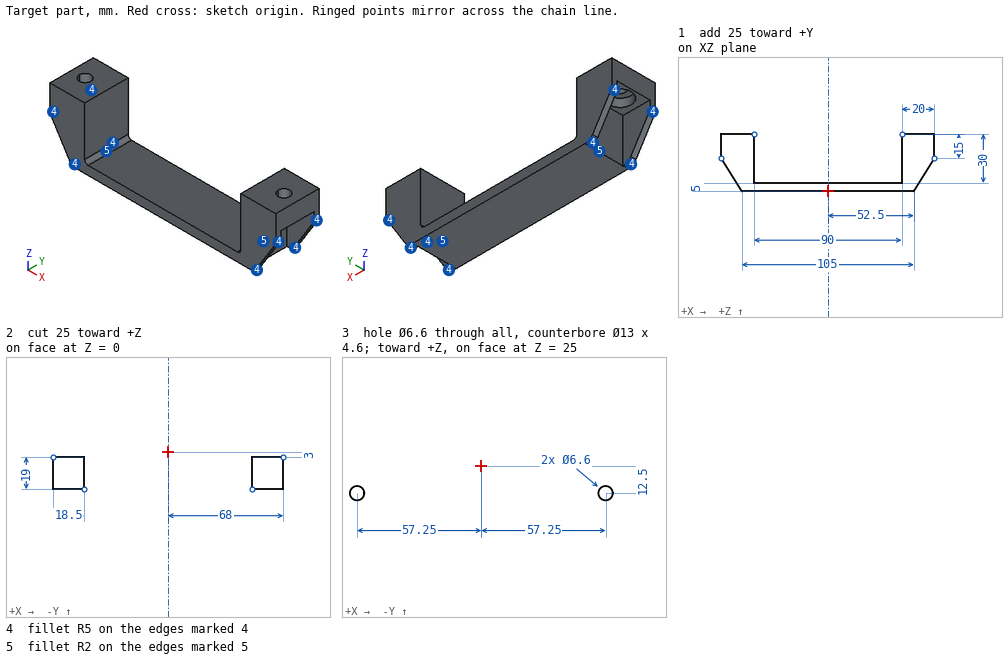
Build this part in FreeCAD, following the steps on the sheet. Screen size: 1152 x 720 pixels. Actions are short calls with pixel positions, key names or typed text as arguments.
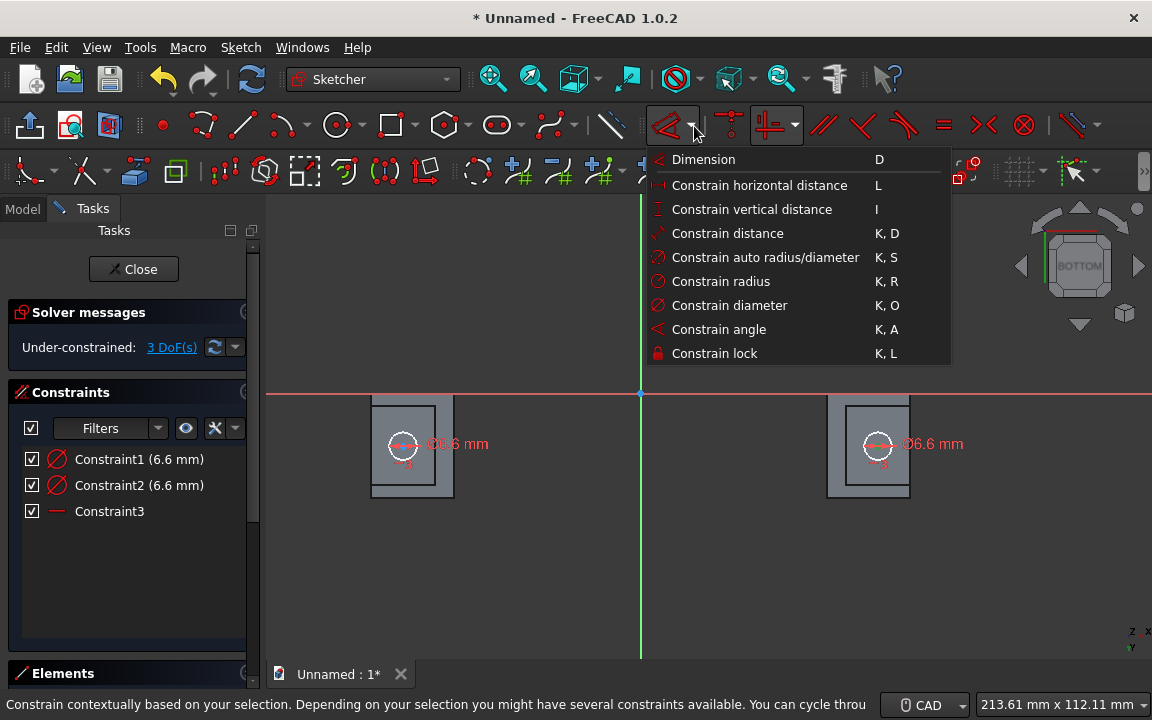
click(799, 209)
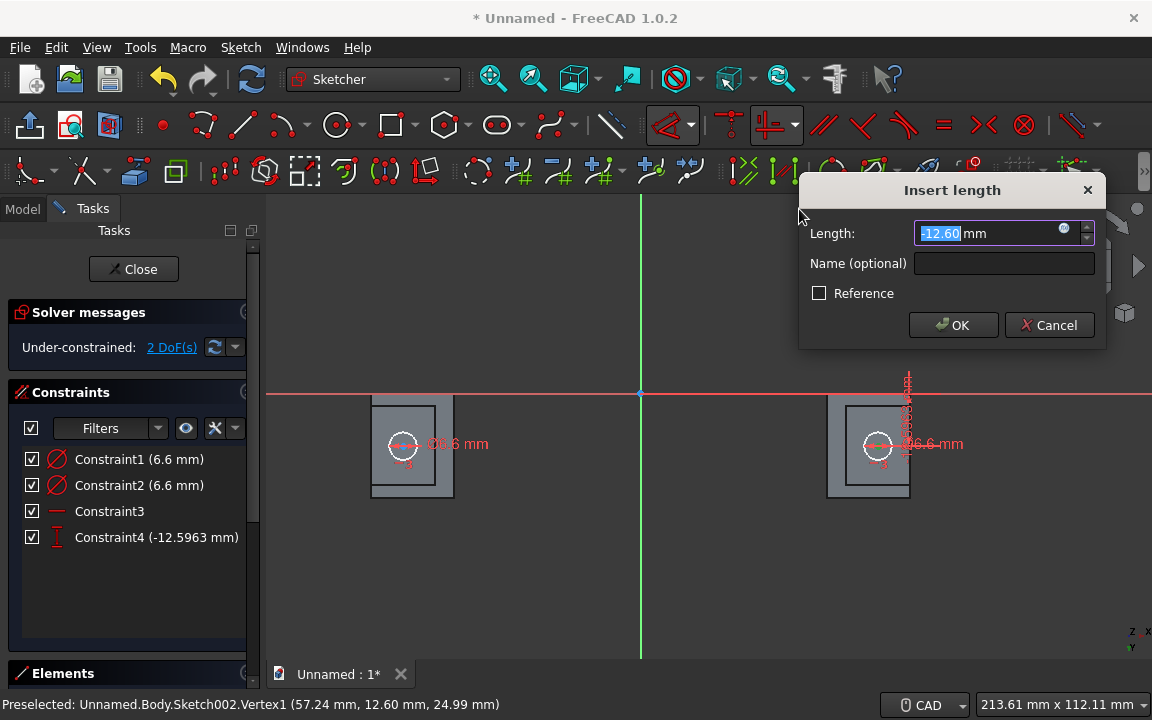
text(-12.5)
key(Return)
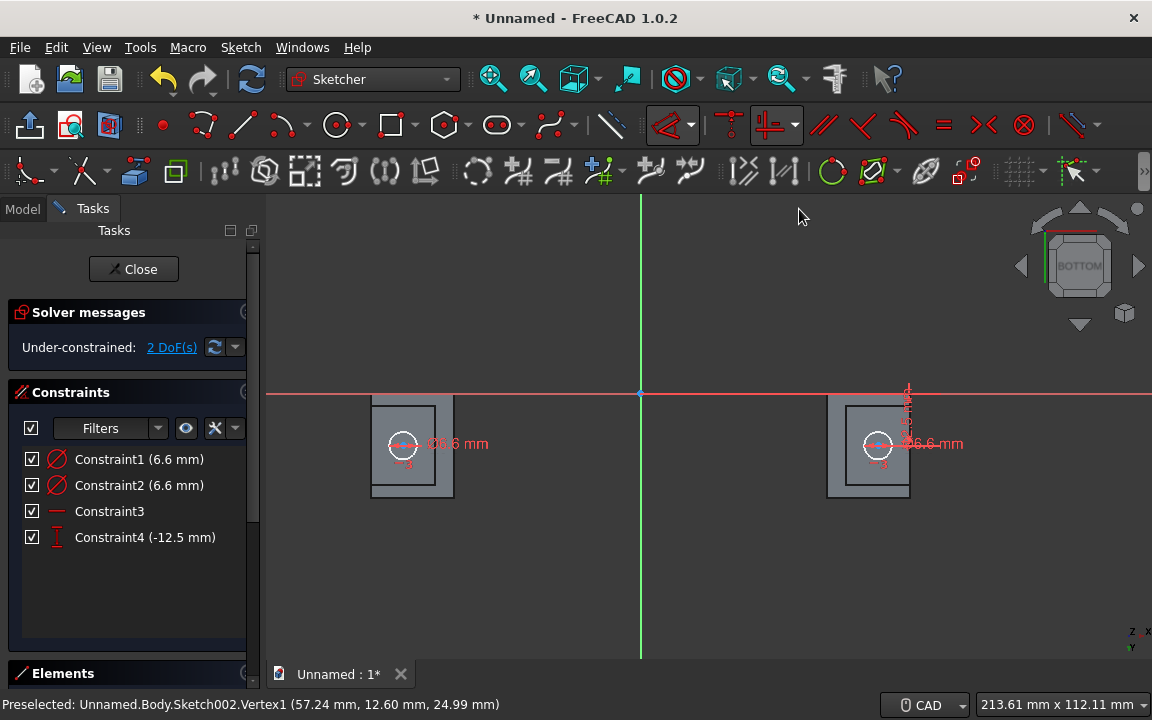
click(878, 446)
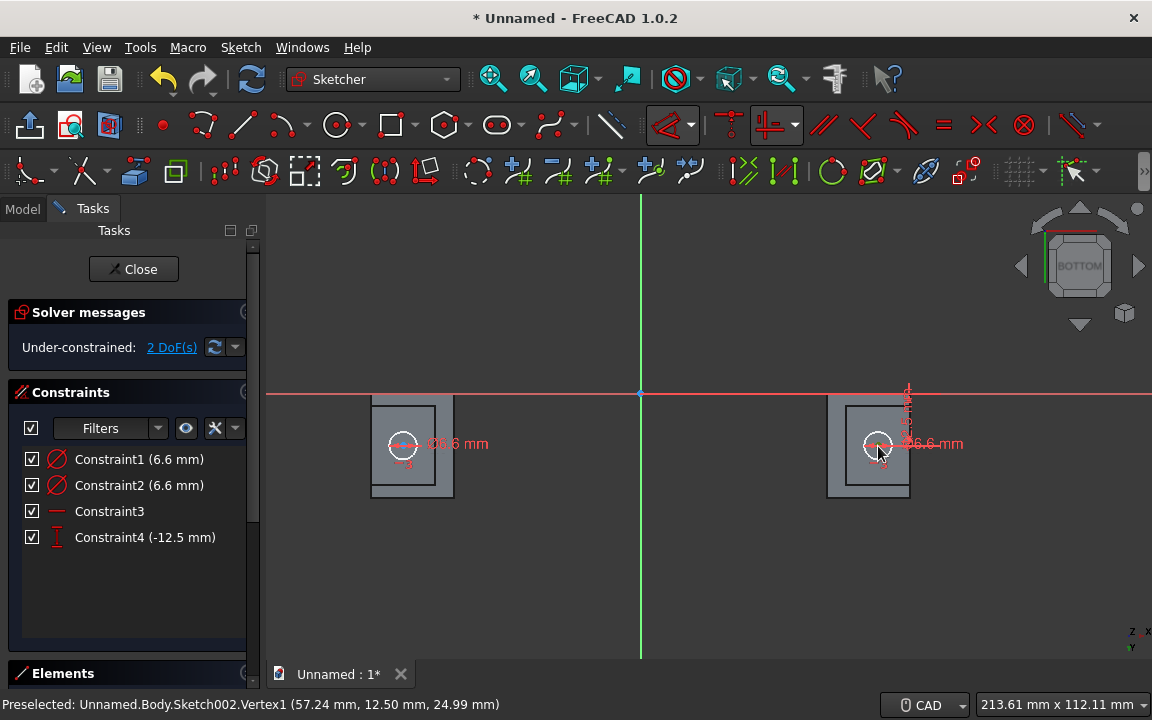
key(l)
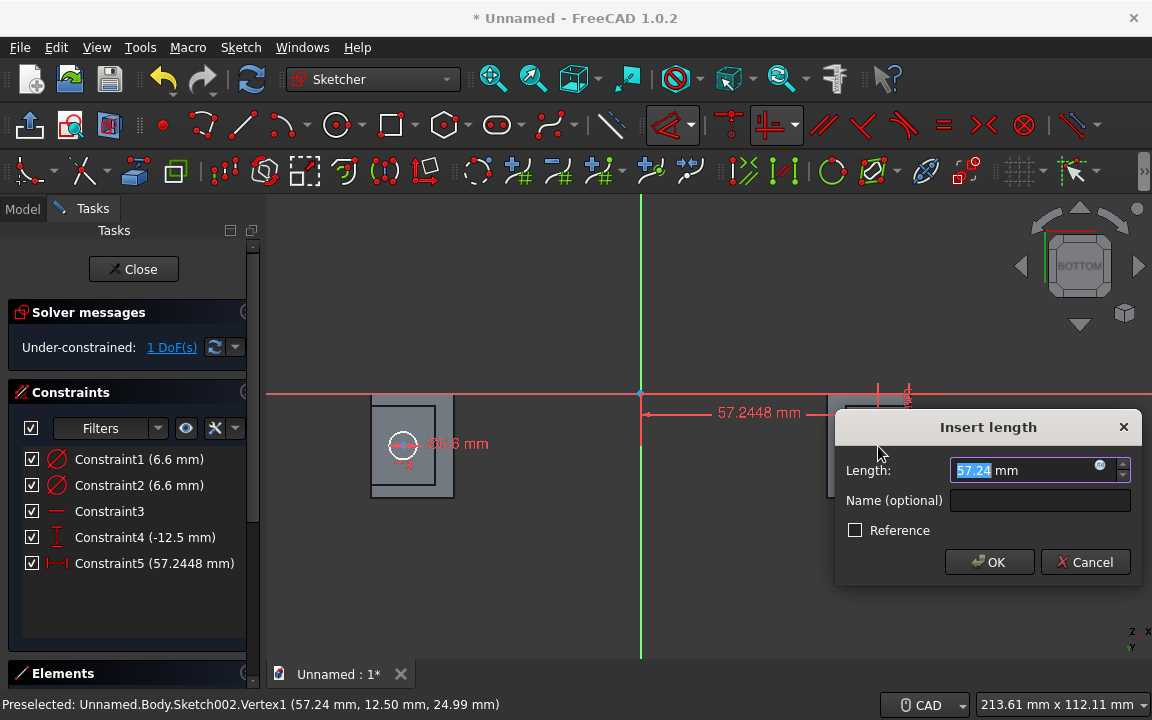
text(57.25)
key(Return)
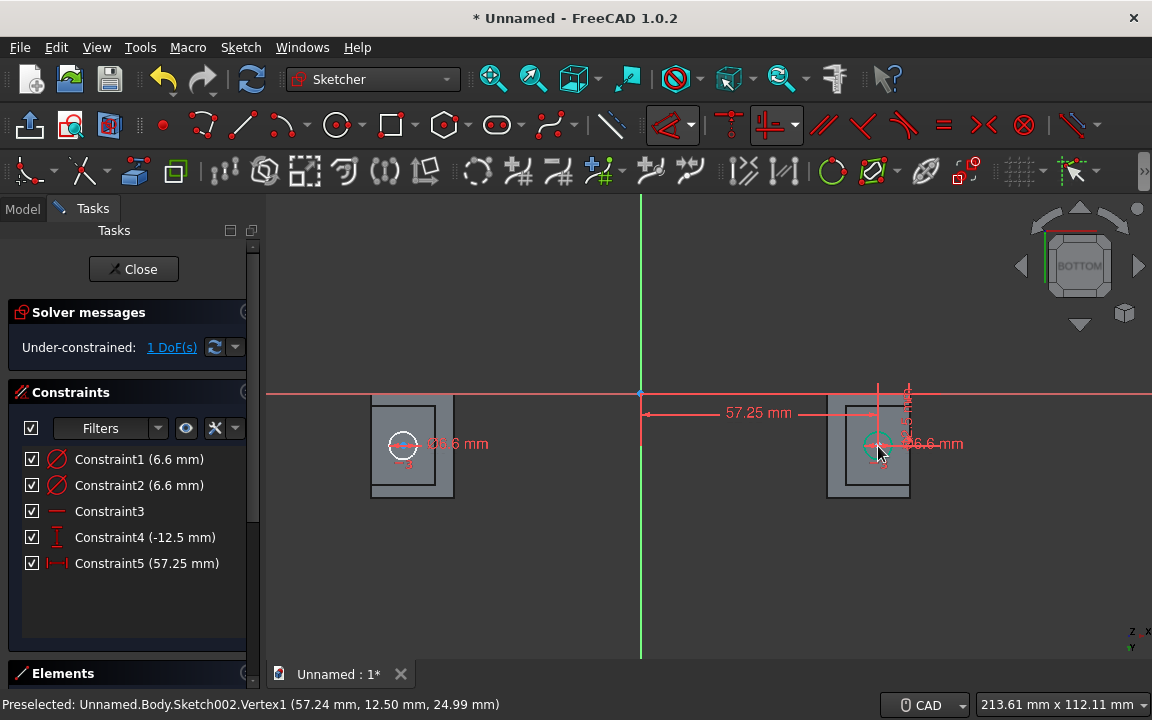
click(403, 446)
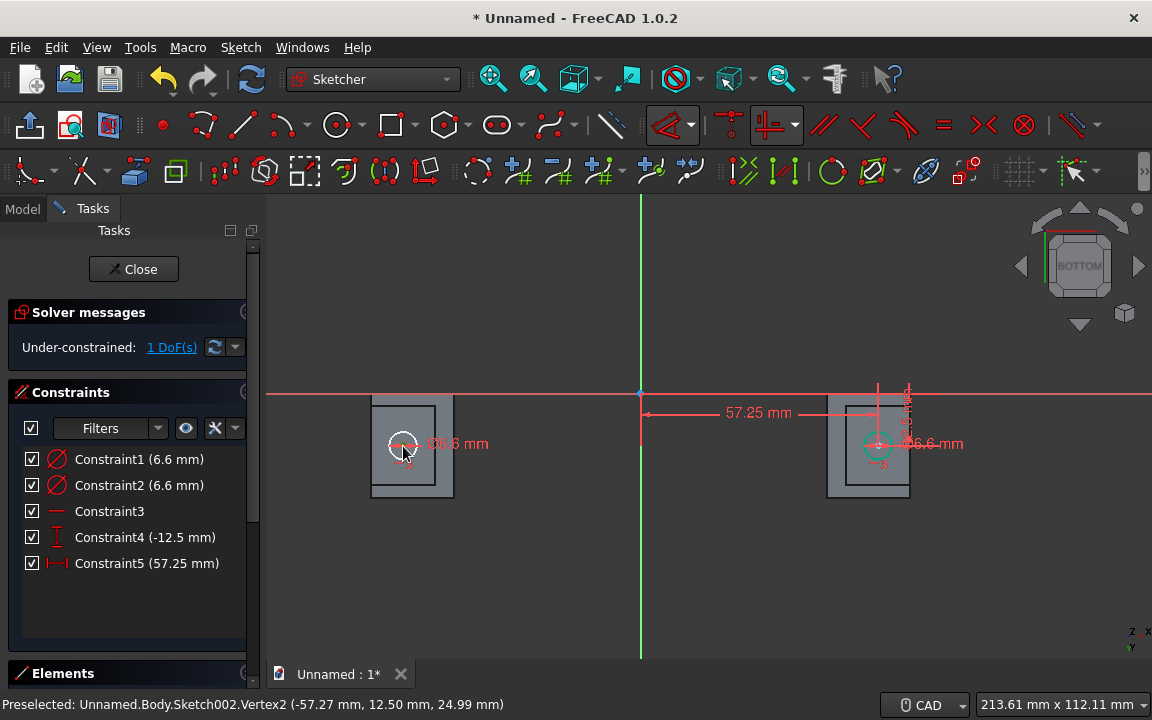
key(l)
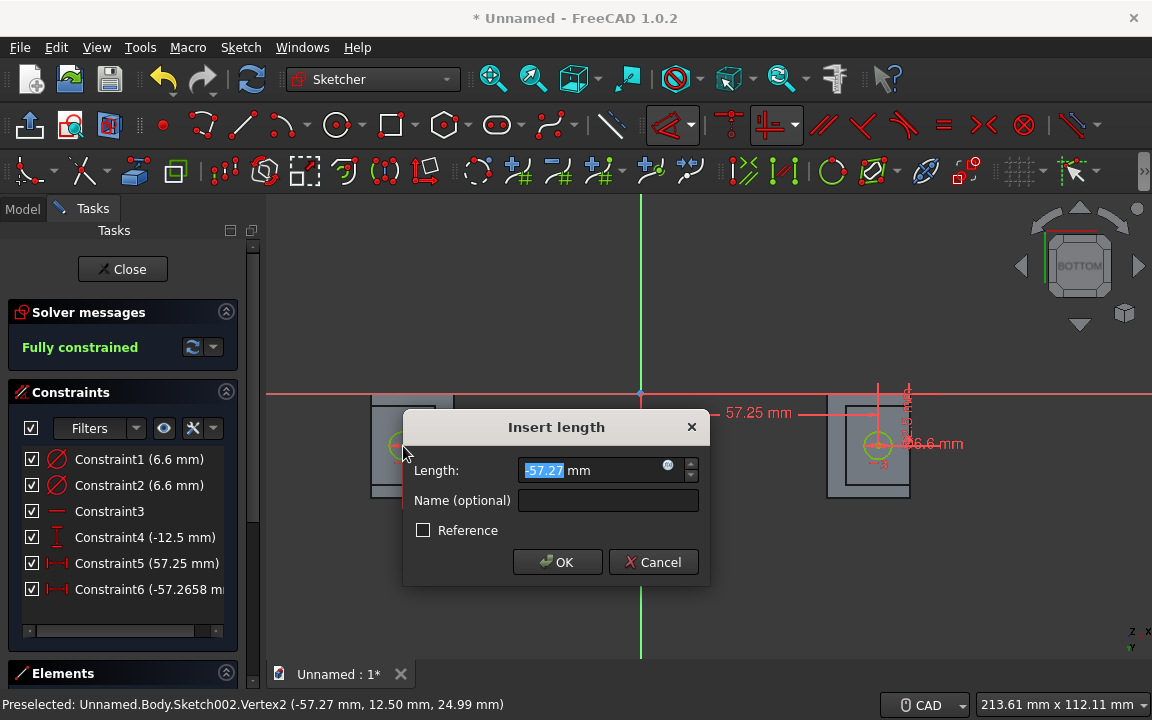
text(-57.25)
key(Return)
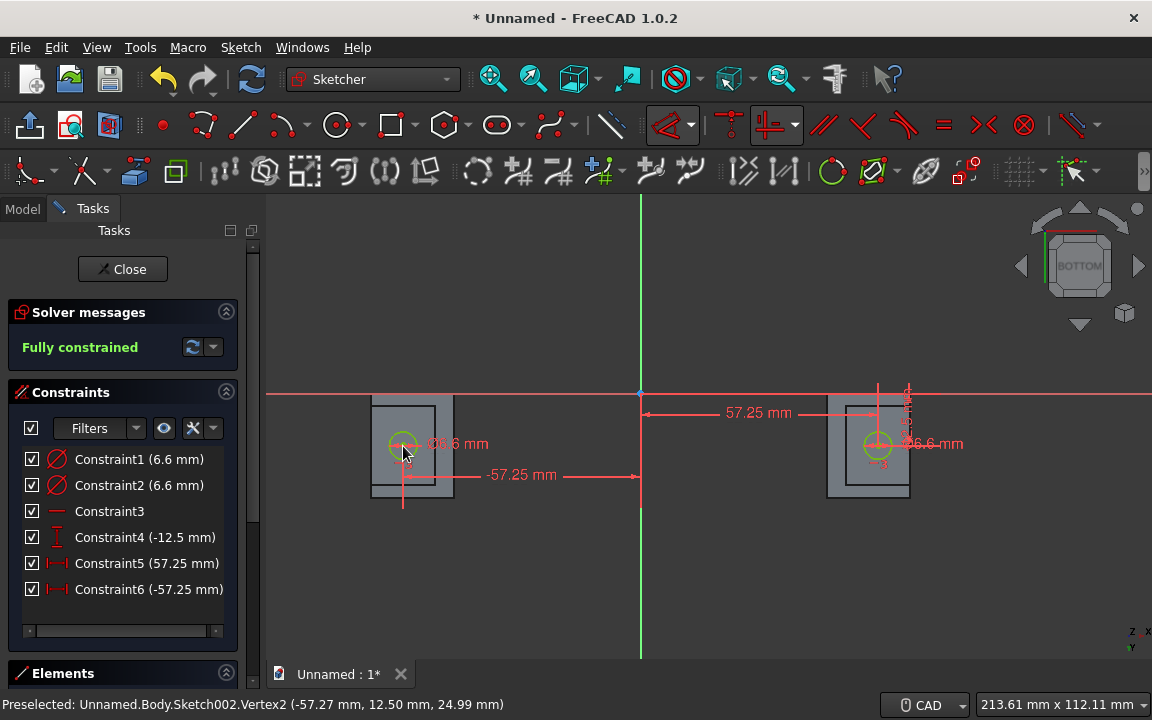
click(123, 269)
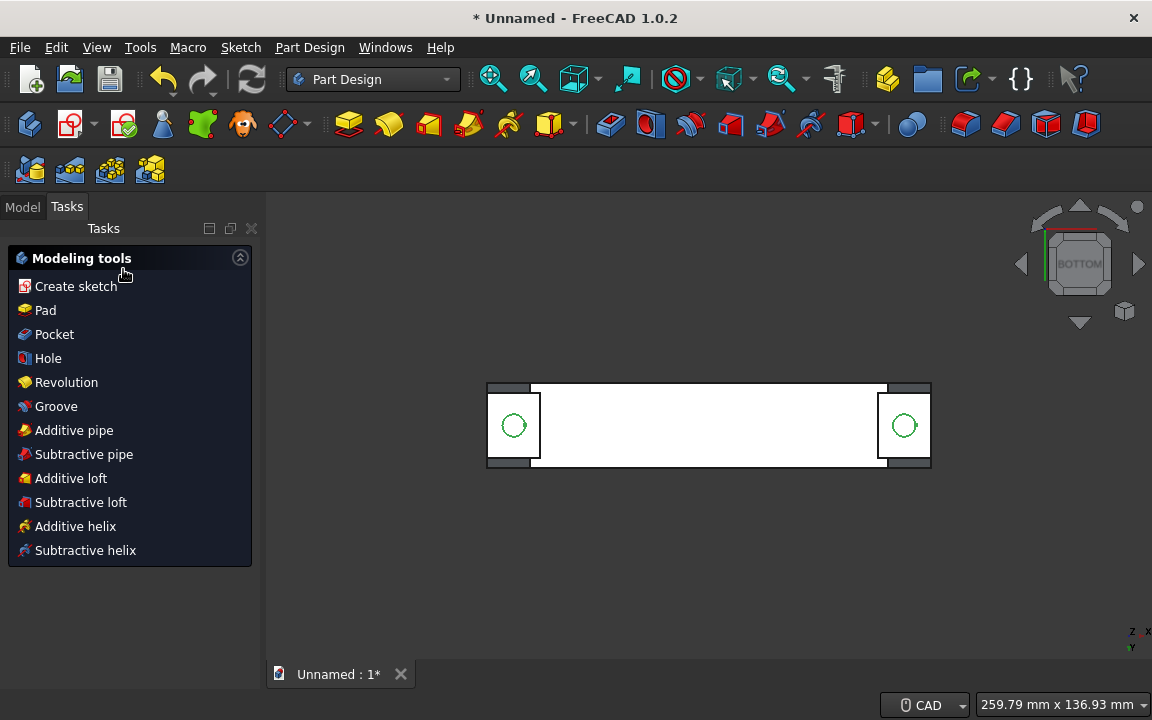
click(652, 124)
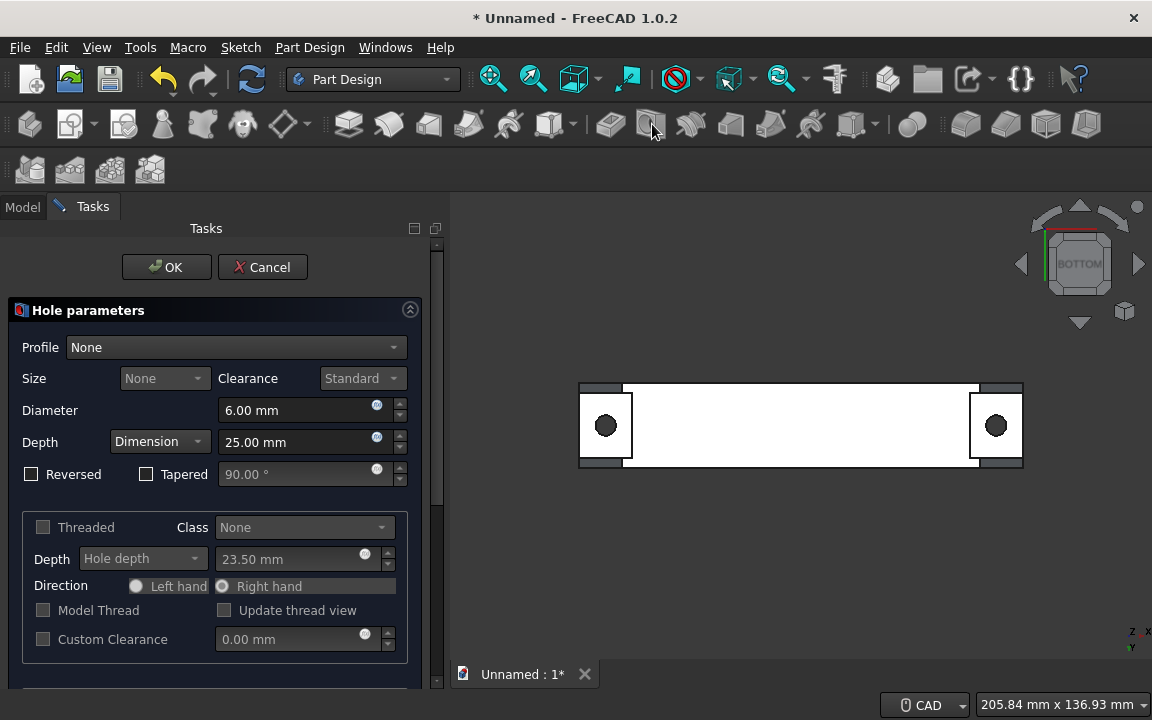
triple_click(305, 410)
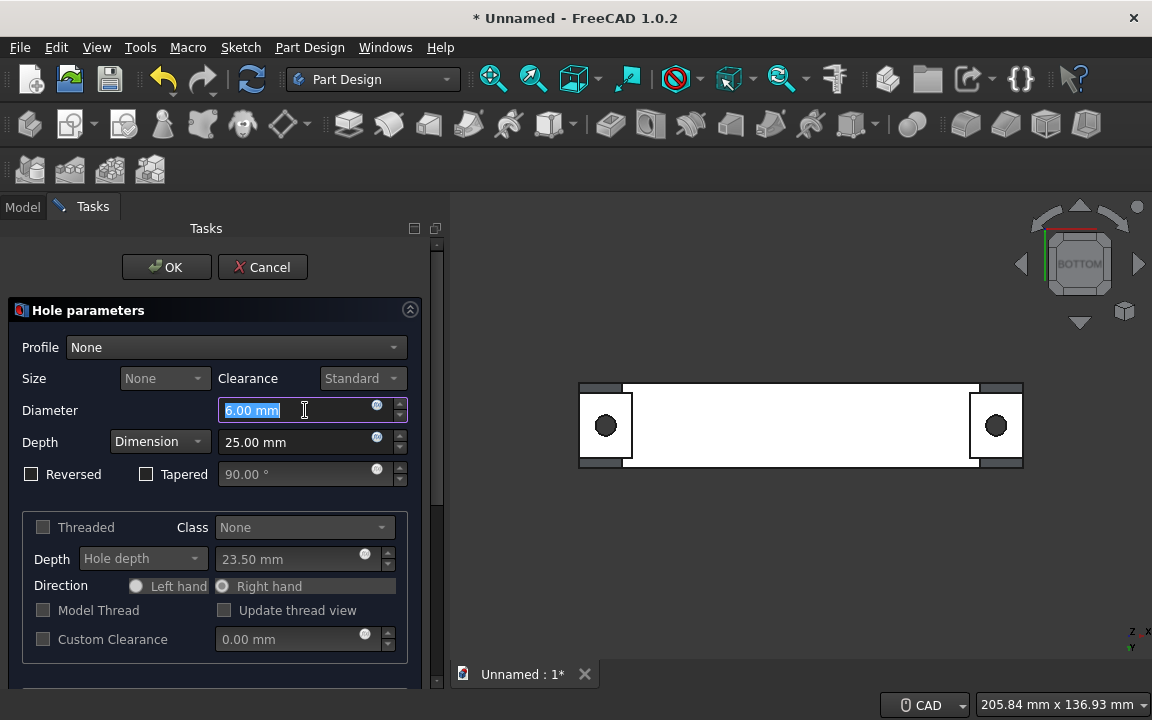
text(6.6)
key(Tab)